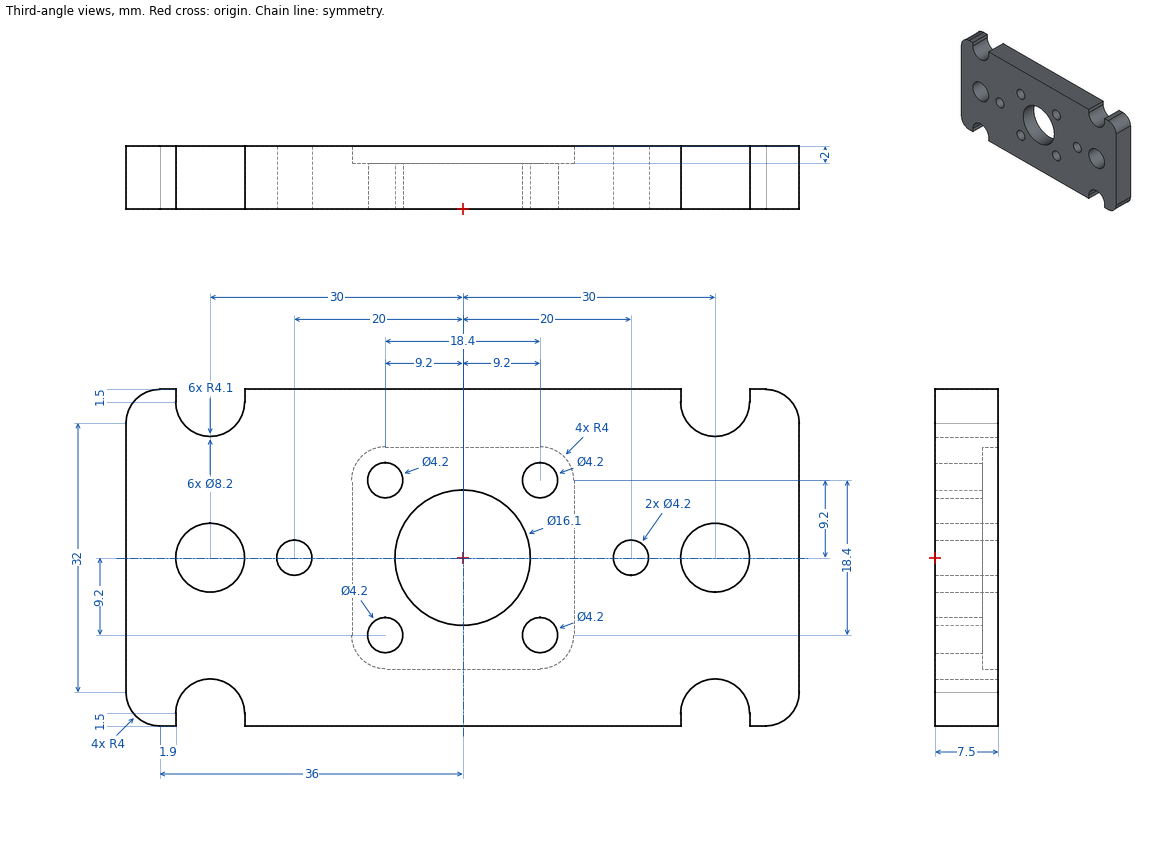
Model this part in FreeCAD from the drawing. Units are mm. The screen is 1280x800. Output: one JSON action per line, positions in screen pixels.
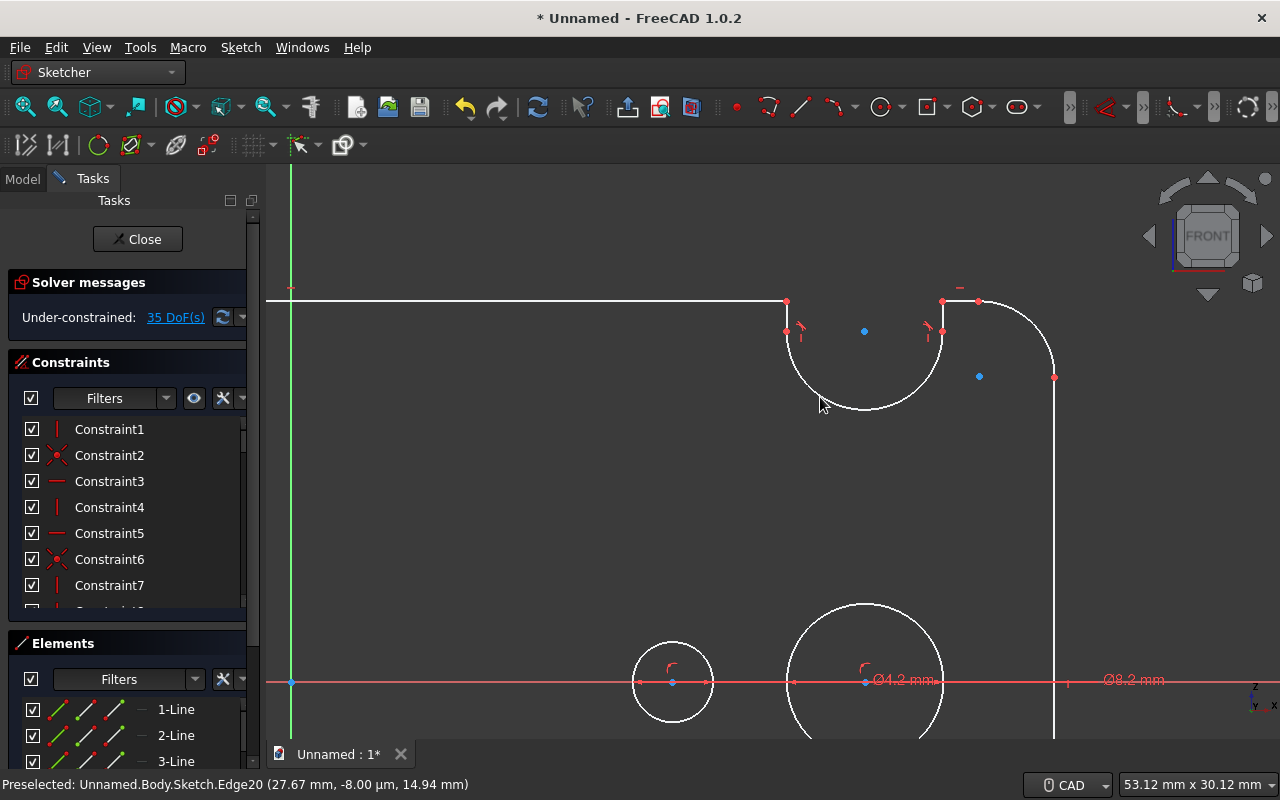
{"action": "scroll", "coordinate": [953, 301], "scroll_direction": "up", "scroll_amount": 2}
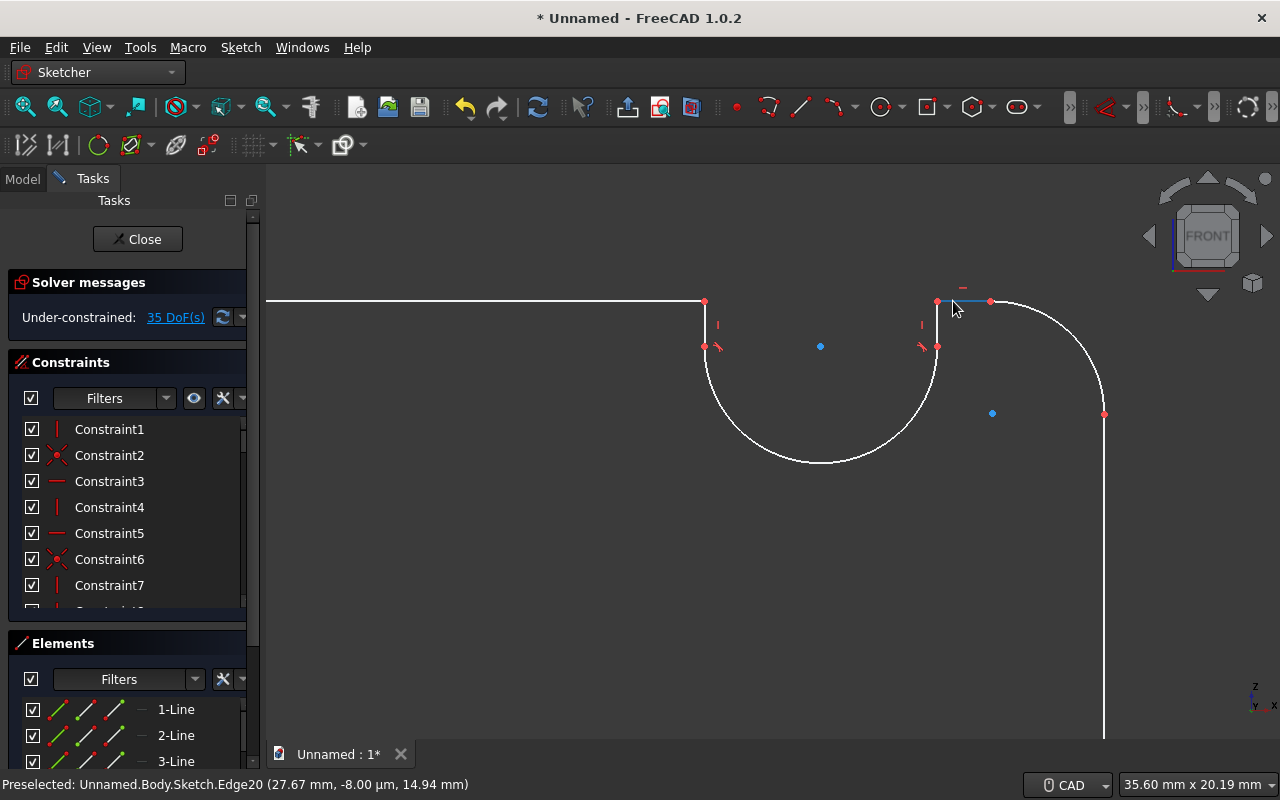
{"action": "left_click", "coordinate": [953, 301]}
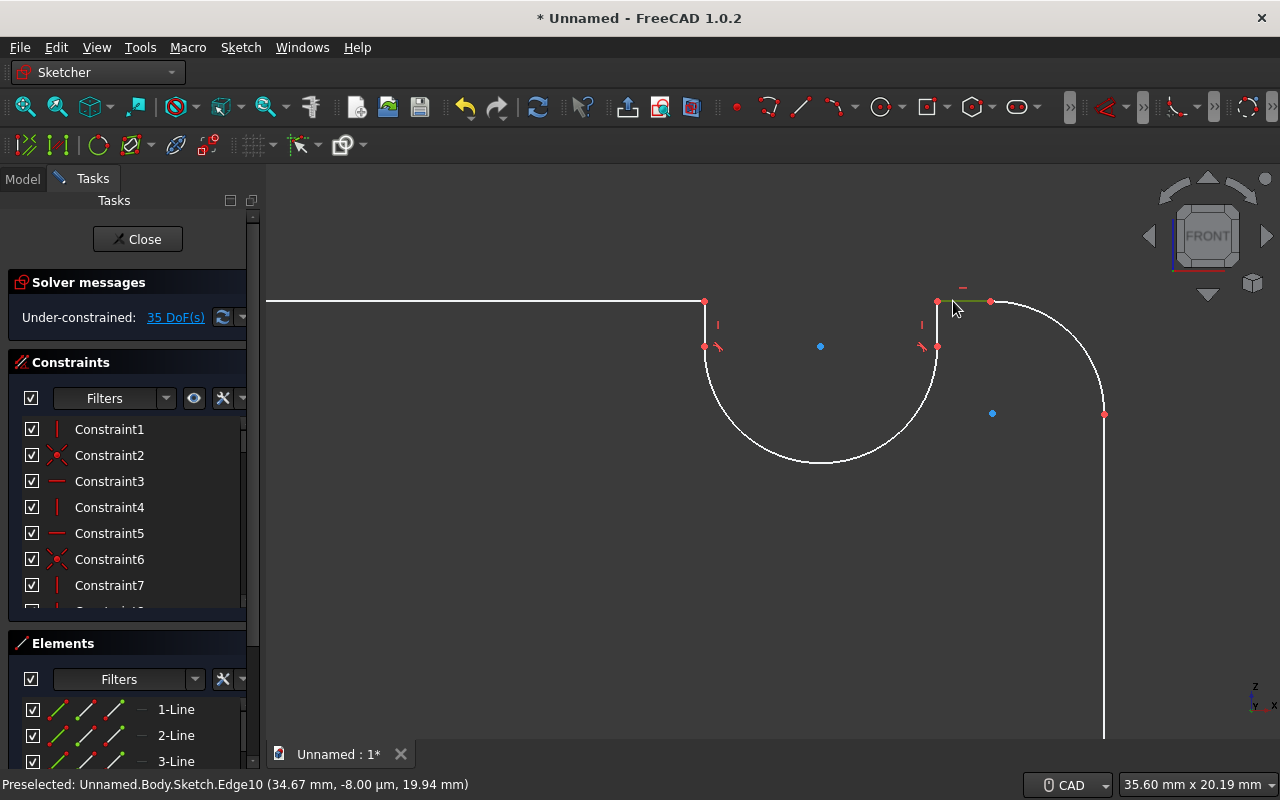
{"action": "scroll", "coordinate": [946, 315], "scroll_direction": "down", "scroll_amount": 7}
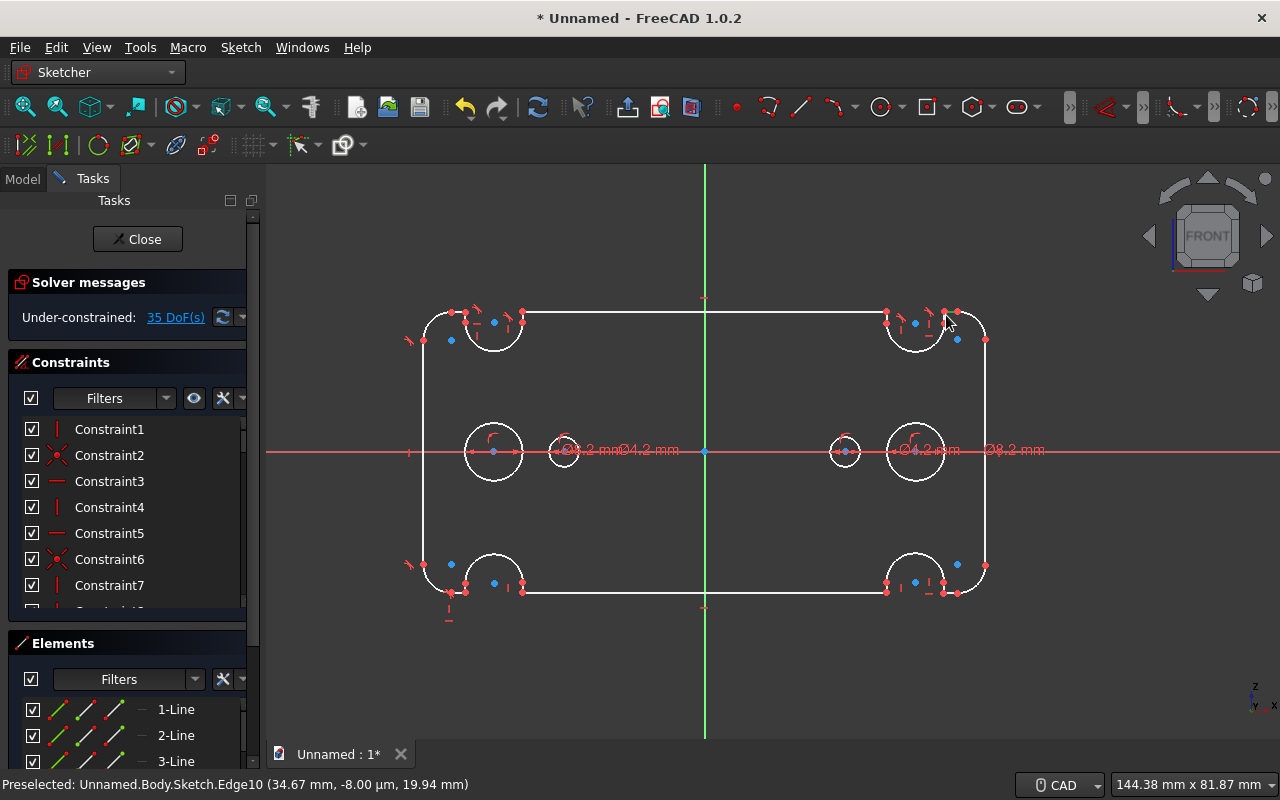
{"action": "left_click", "coordinate": [983, 327]}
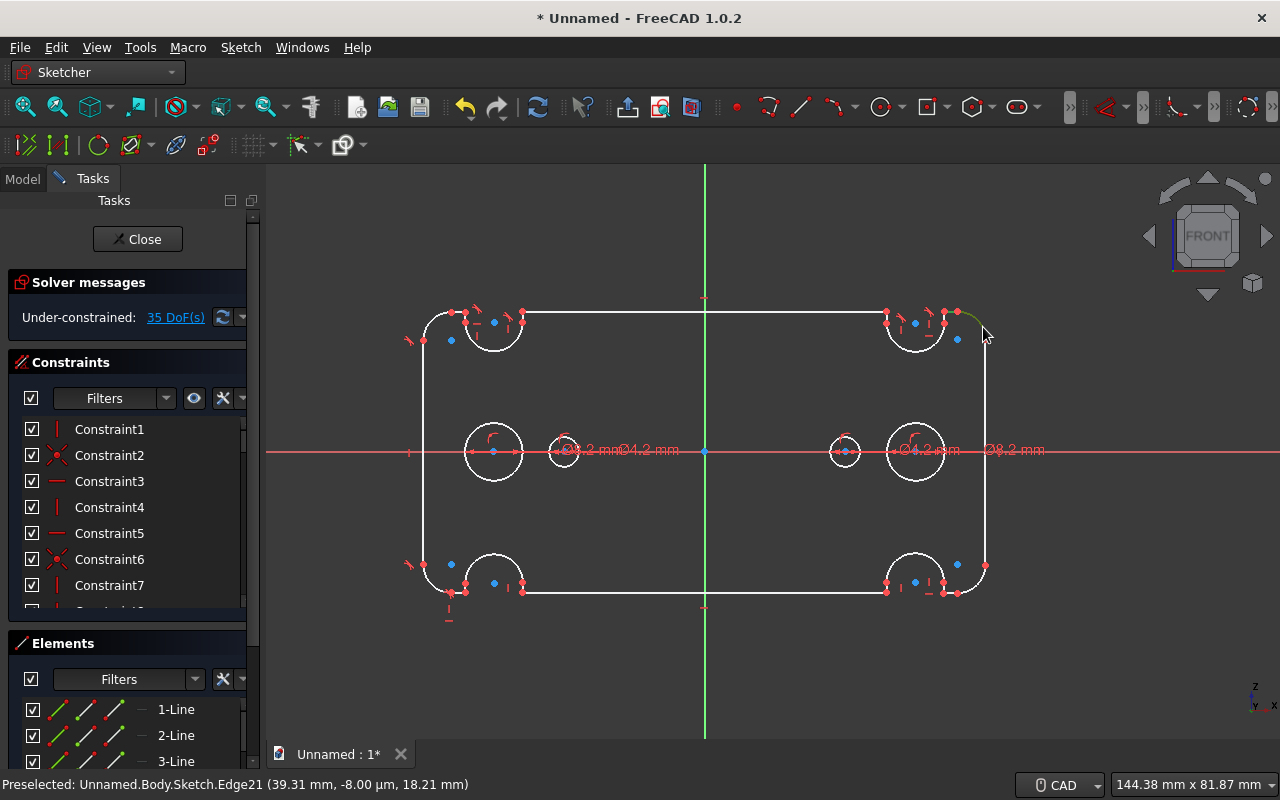
{"action": "key", "text": "t"}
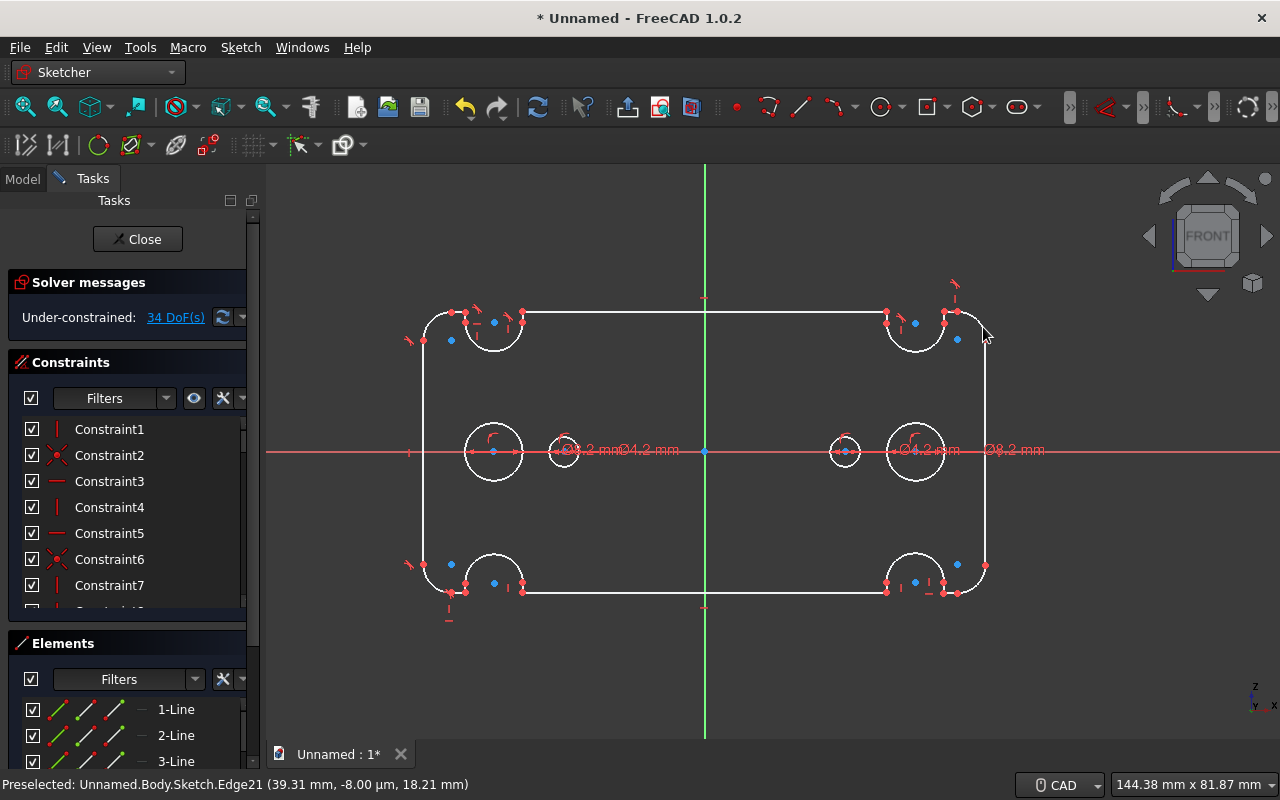
{"action": "left_click", "coordinate": [985, 407]}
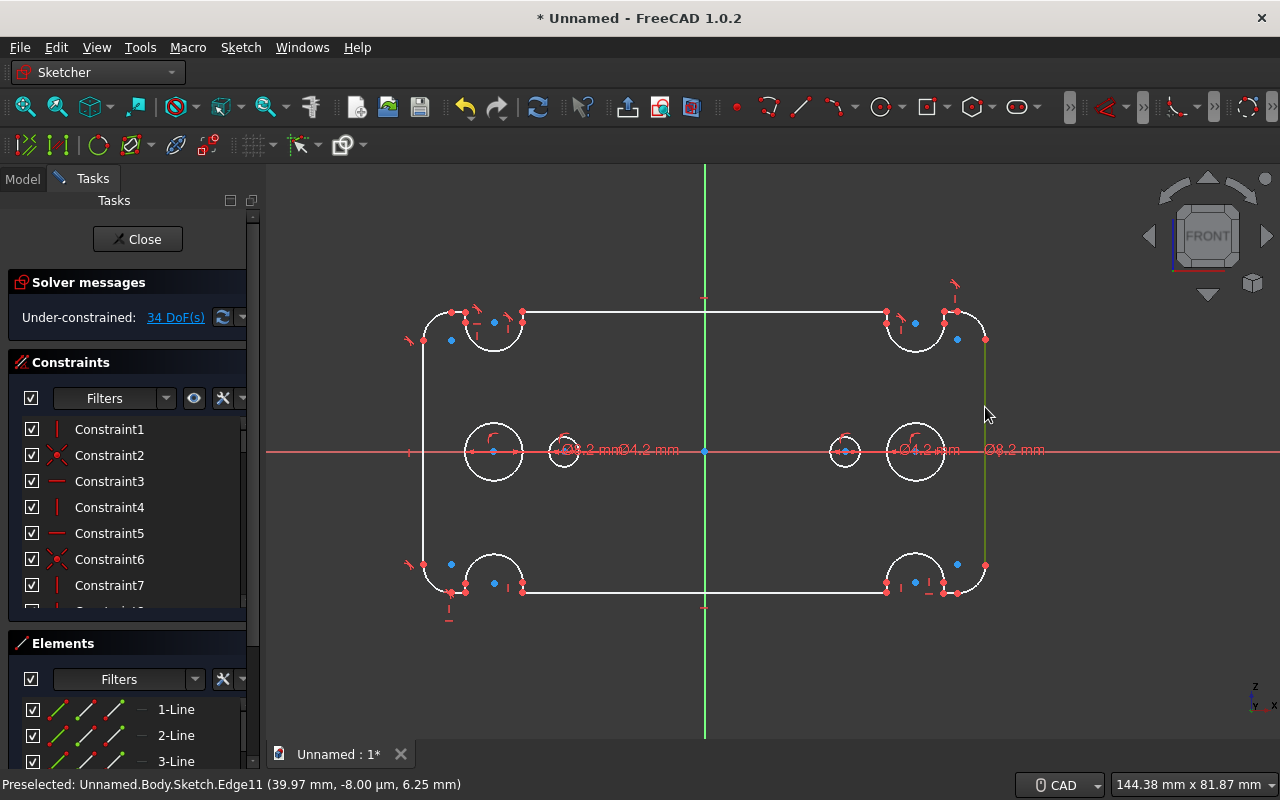
{"action": "left_click", "coordinate": [982, 327]}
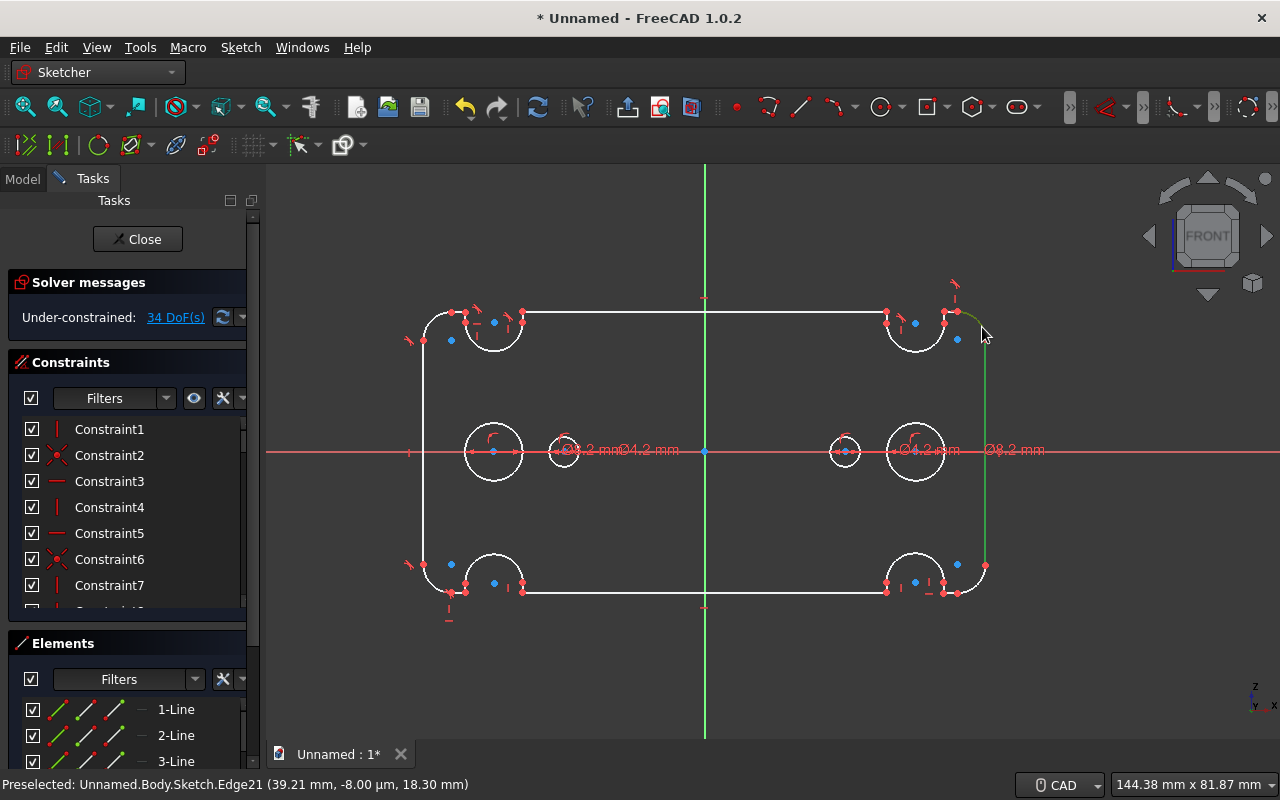
{"action": "key", "text": "t"}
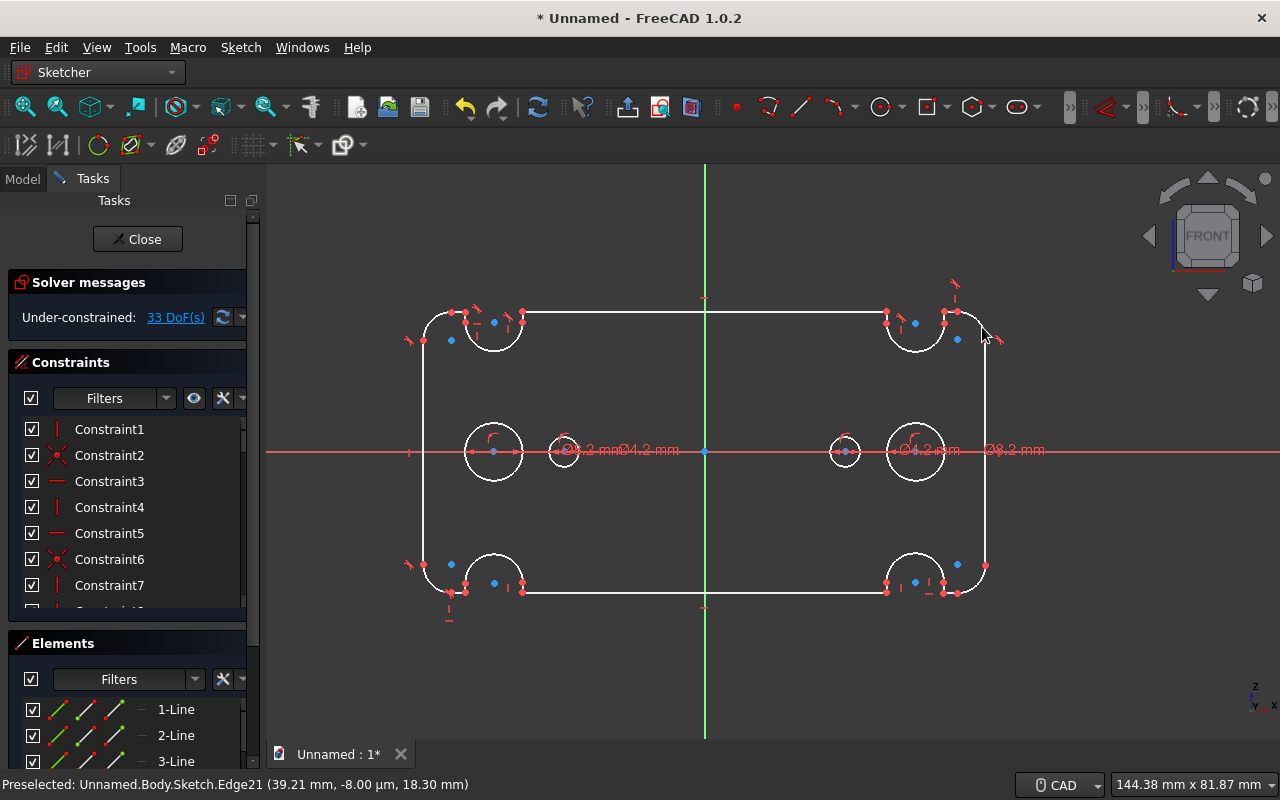
{"action": "left_click", "coordinate": [985, 407]}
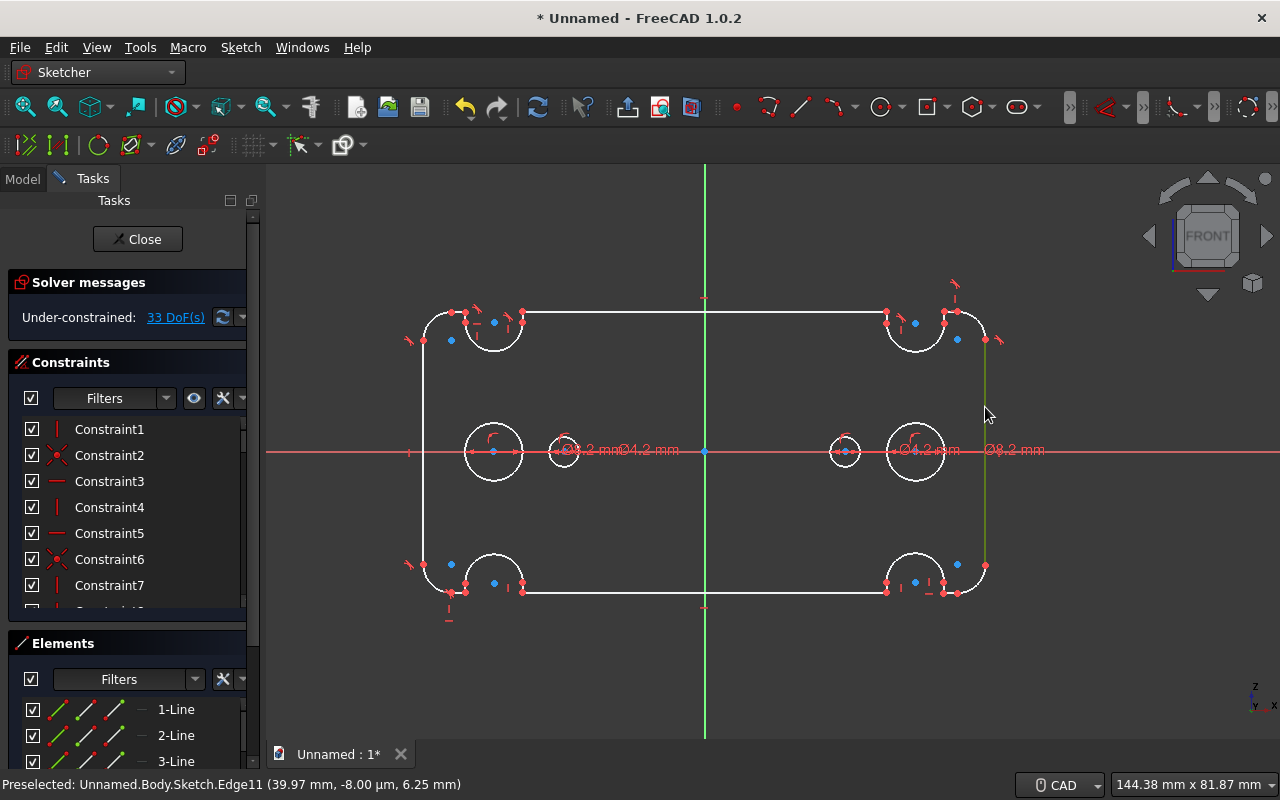
{"action": "left_click", "coordinate": [970, 590]}